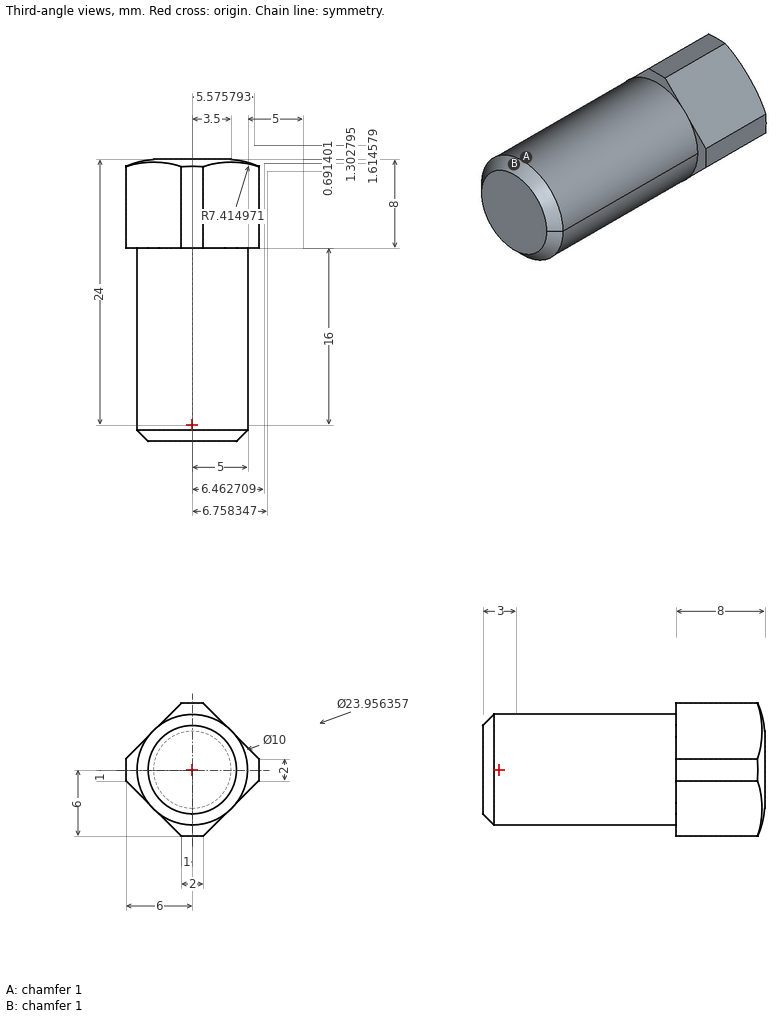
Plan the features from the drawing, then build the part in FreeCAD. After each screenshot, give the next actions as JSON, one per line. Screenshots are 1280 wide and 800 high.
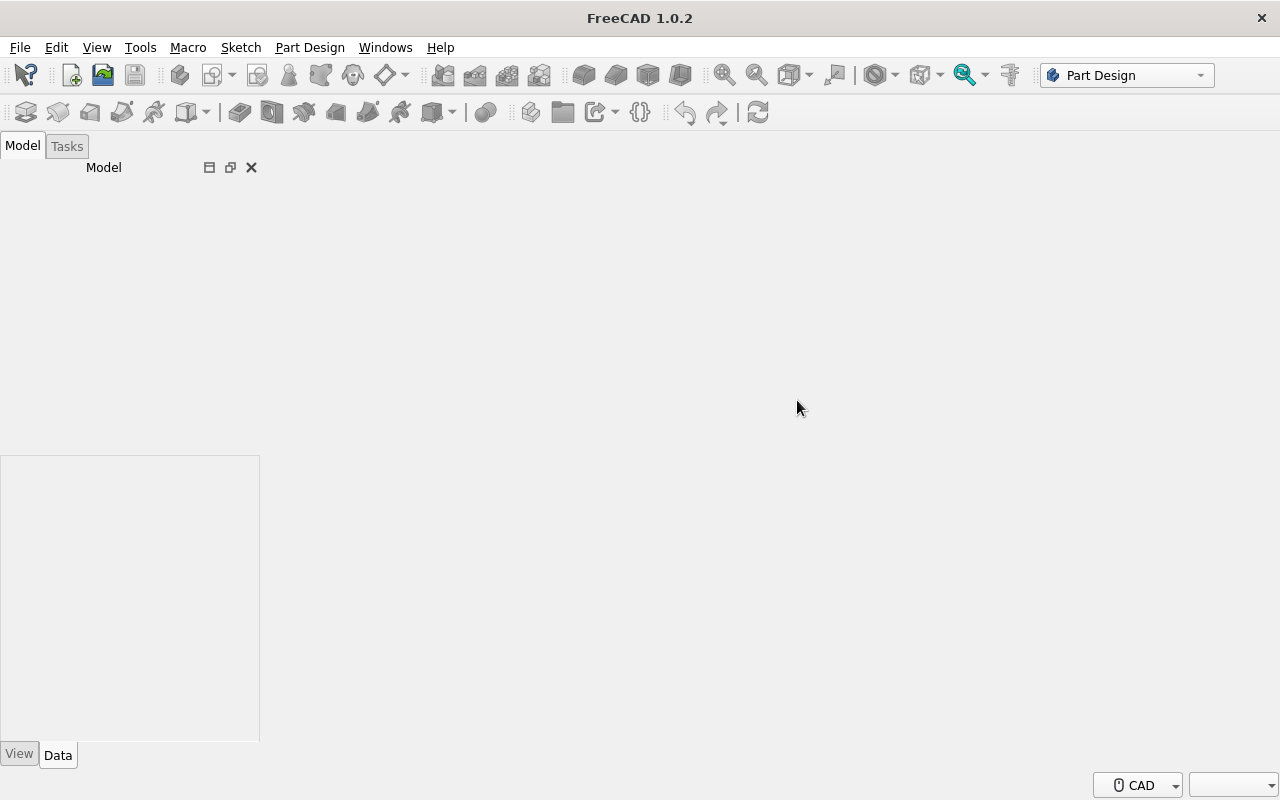
{"action": "key", "text": "ctrl+n"}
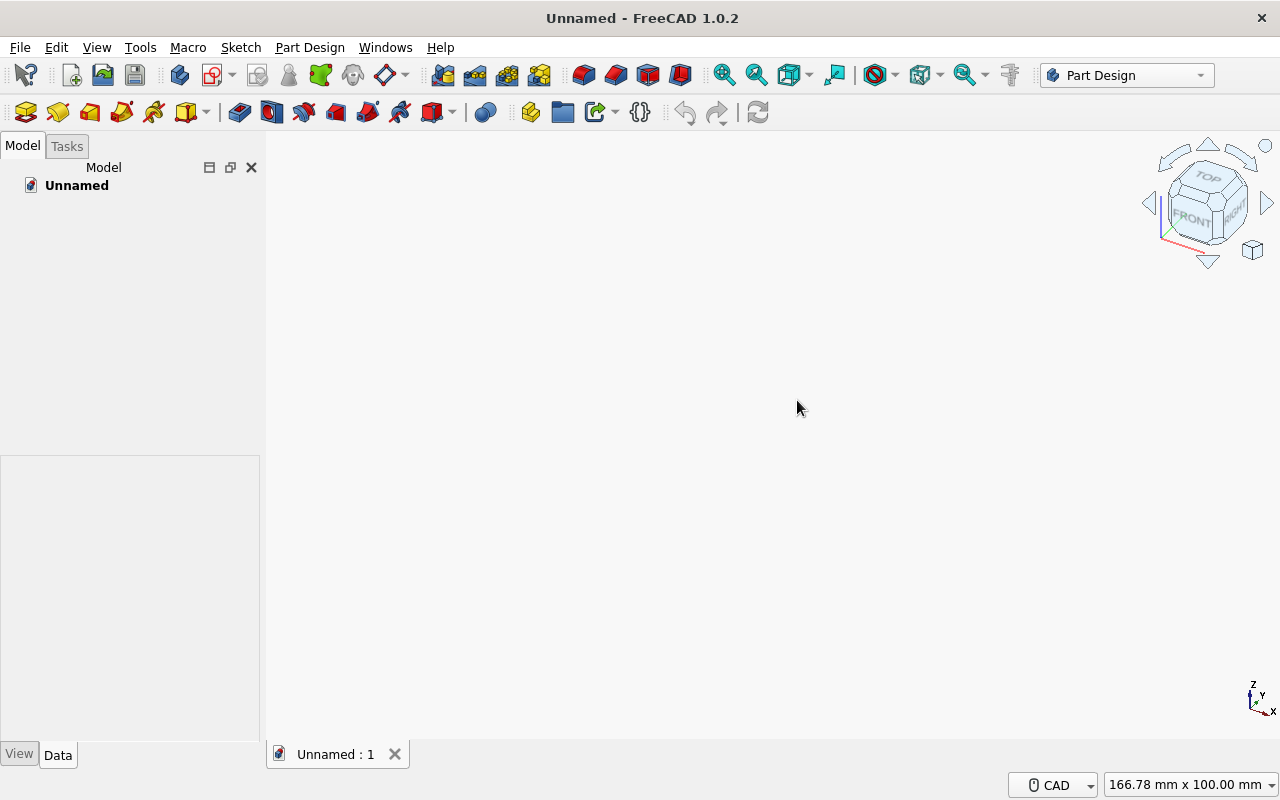
{"action": "left_click", "coordinate": [212, 76]}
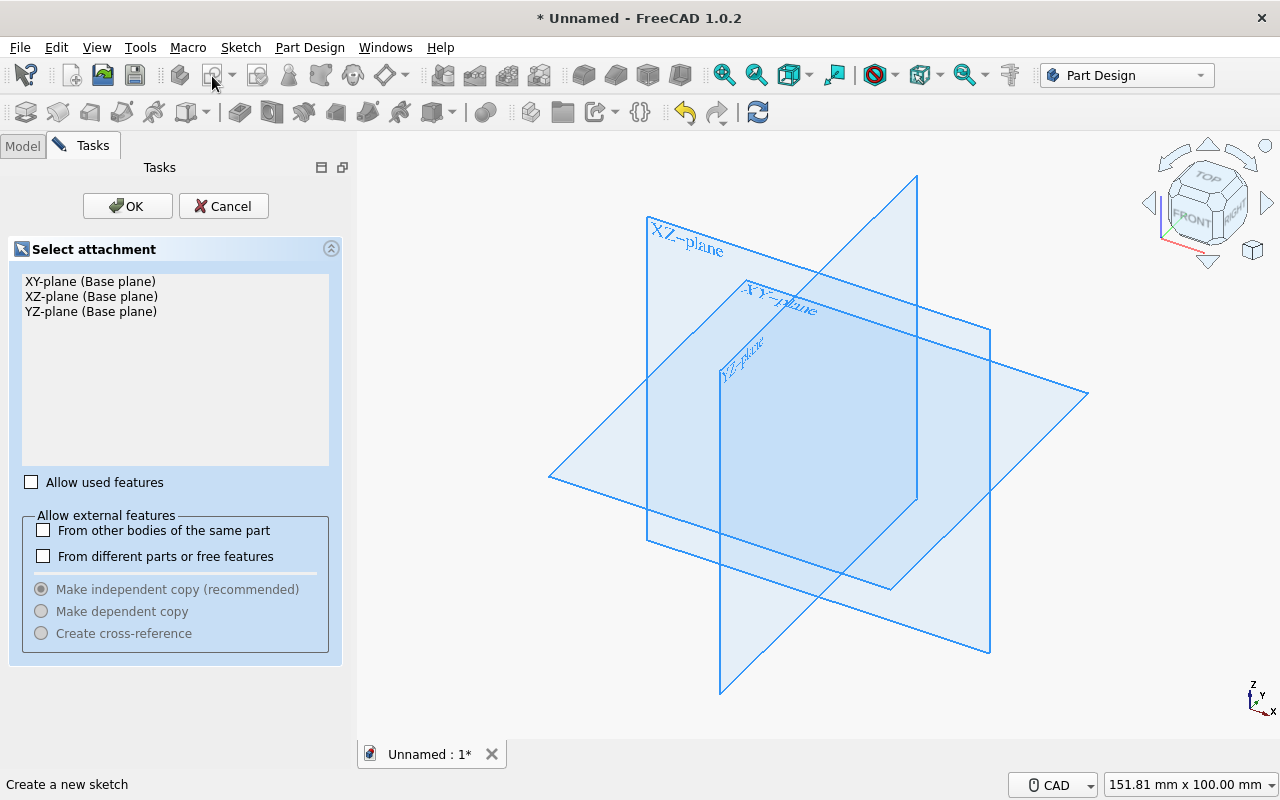
{"action": "left_click", "coordinate": [82, 282]}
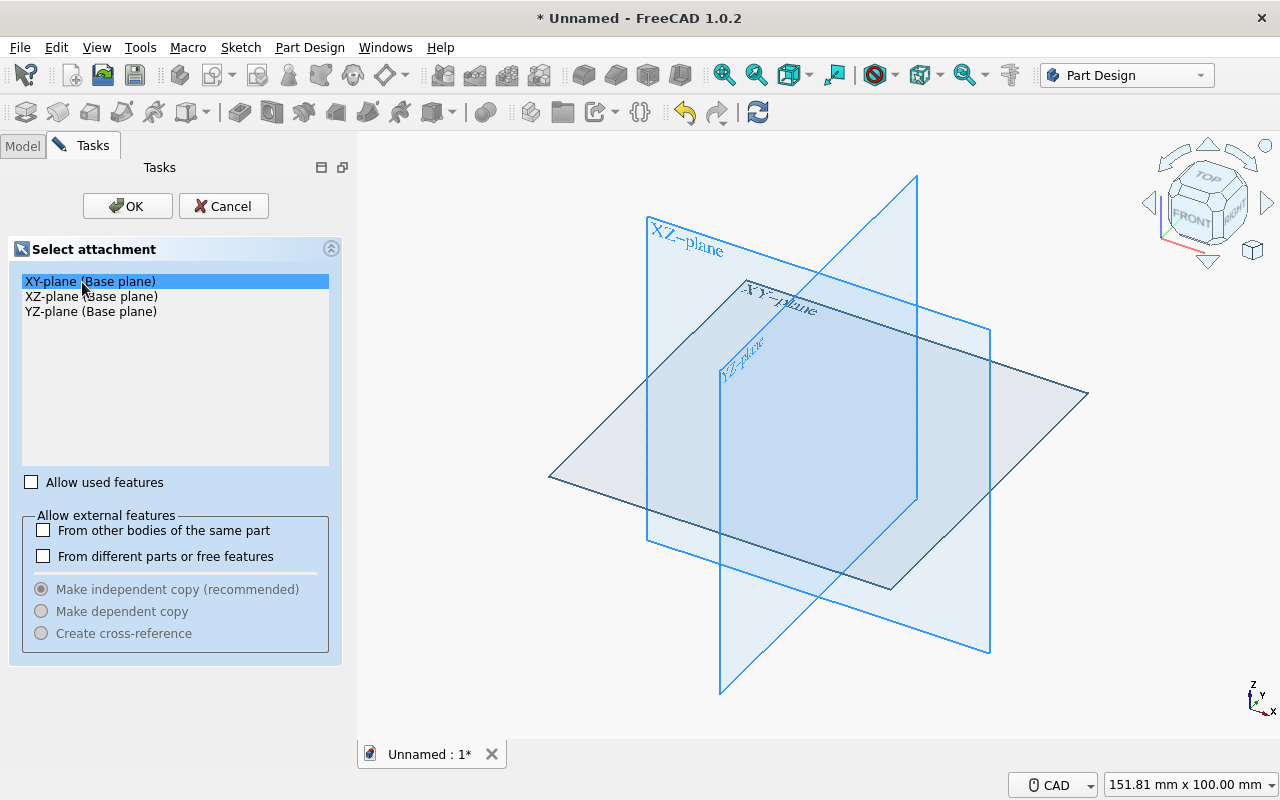
{"action": "left_click", "coordinate": [128, 206]}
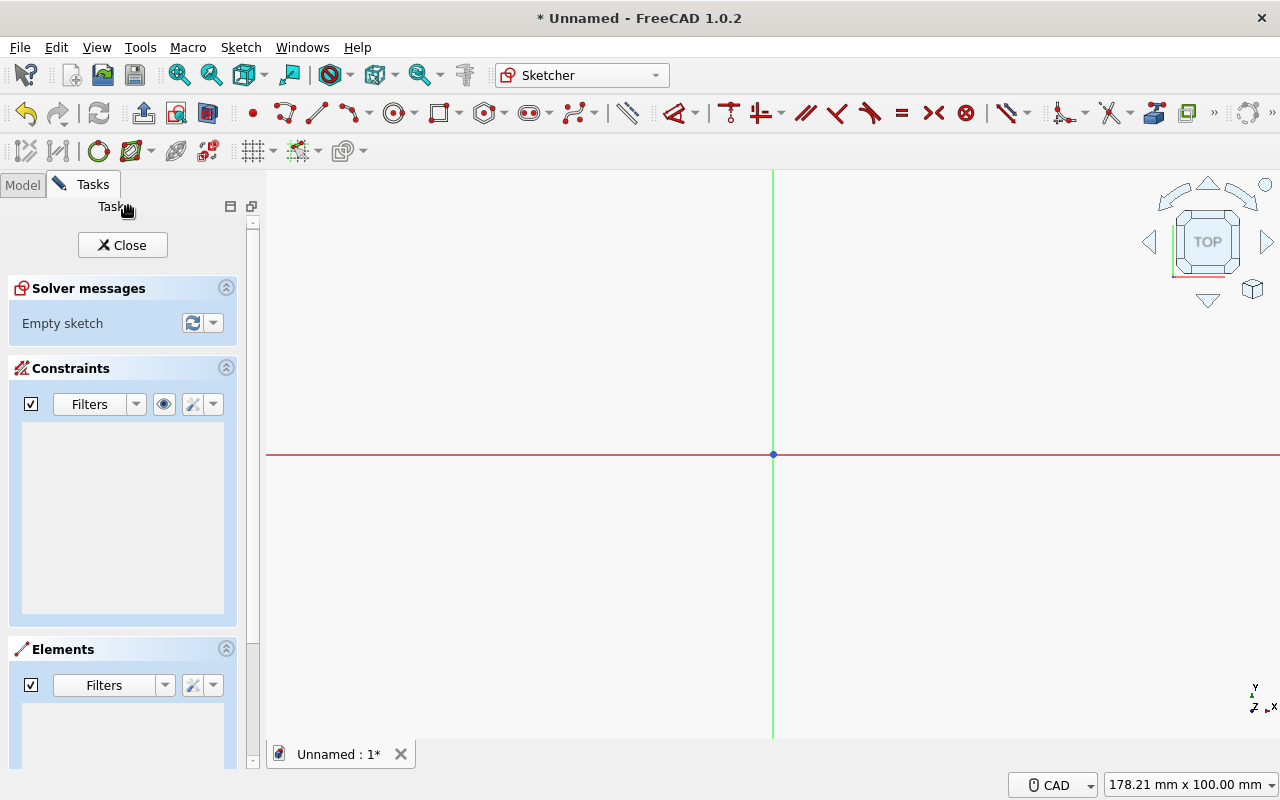
{"action": "scroll", "coordinate": [858, 346], "scroll_direction": "up", "scroll_amount": 5}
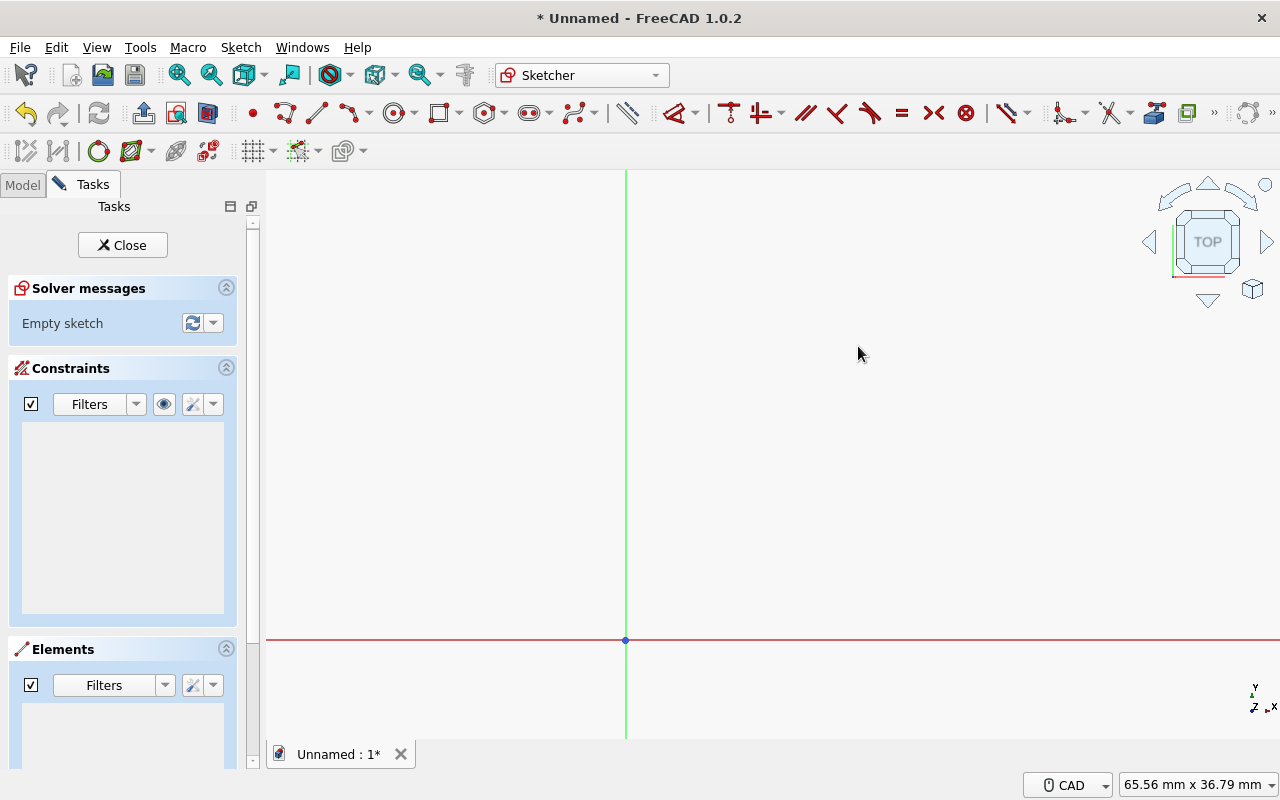
{"action": "left_click", "coordinate": [286, 114]}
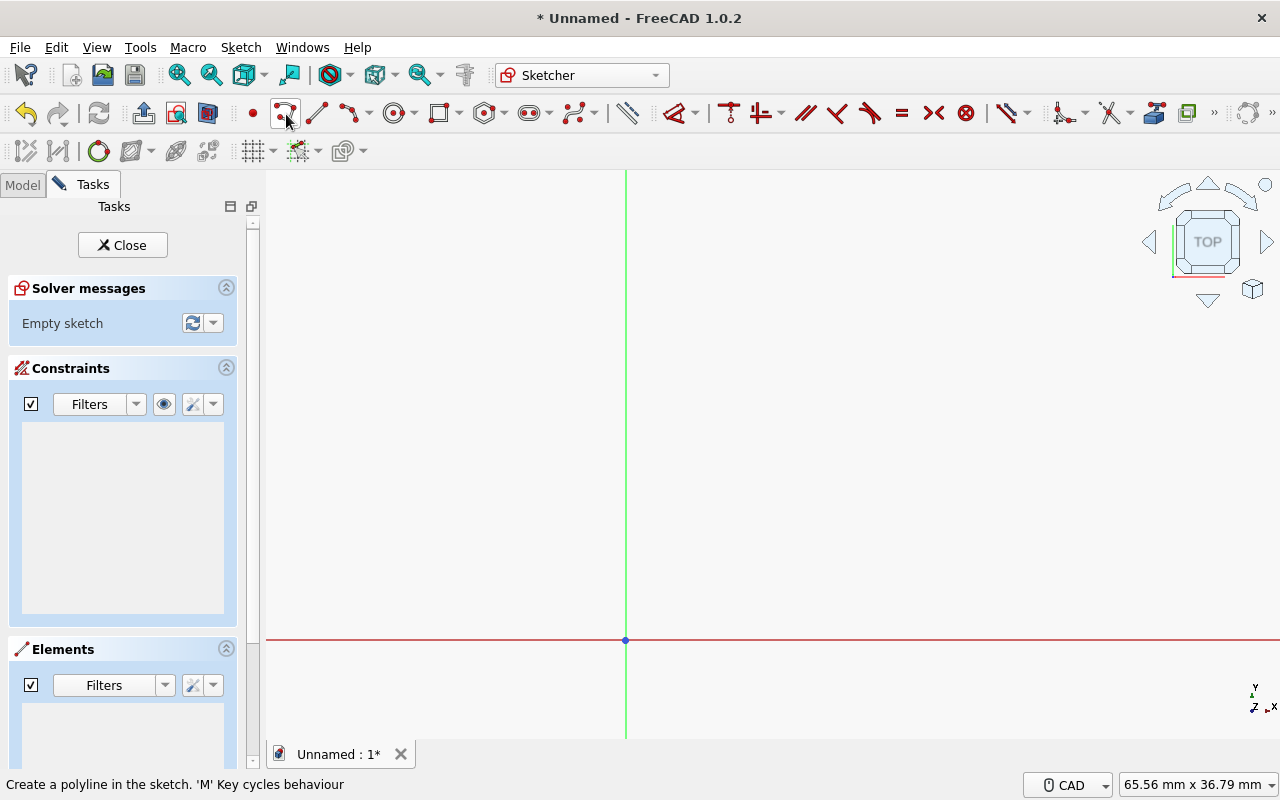
{"action": "left_click", "coordinate": [626, 640]}
{"action": "left_click", "coordinate": [703, 631]}
{"action": "left_click", "coordinate": [703, 393]}
{"action": "left_click", "coordinate": [781, 393]}
{"action": "left_click", "coordinate": [781, 269]}
{"action": "left_click", "coordinate": [635, 269]}
{"action": "left_click", "coordinate": [626, 640]}
{"action": "key", "text": "Escape"}
{"action": "key", "text": "Escape"}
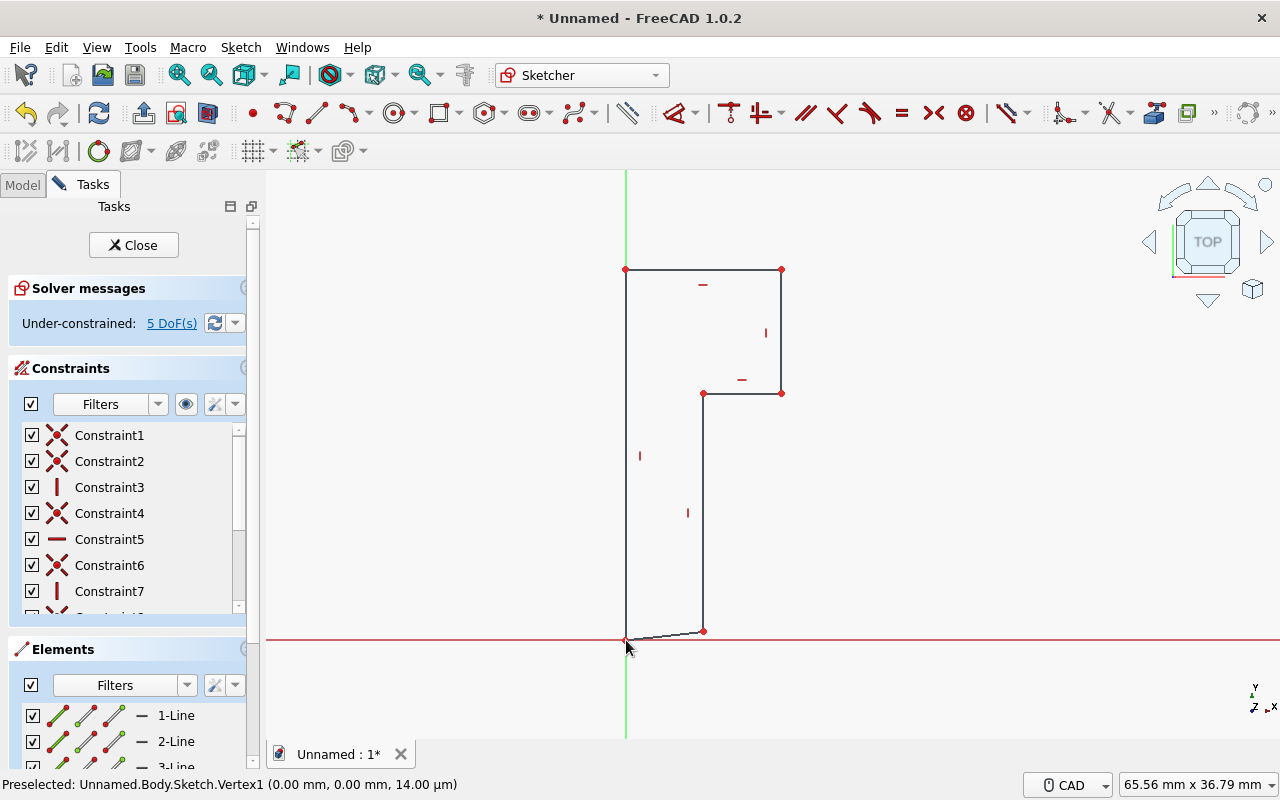
{"action": "left_click", "coordinate": [649, 638]}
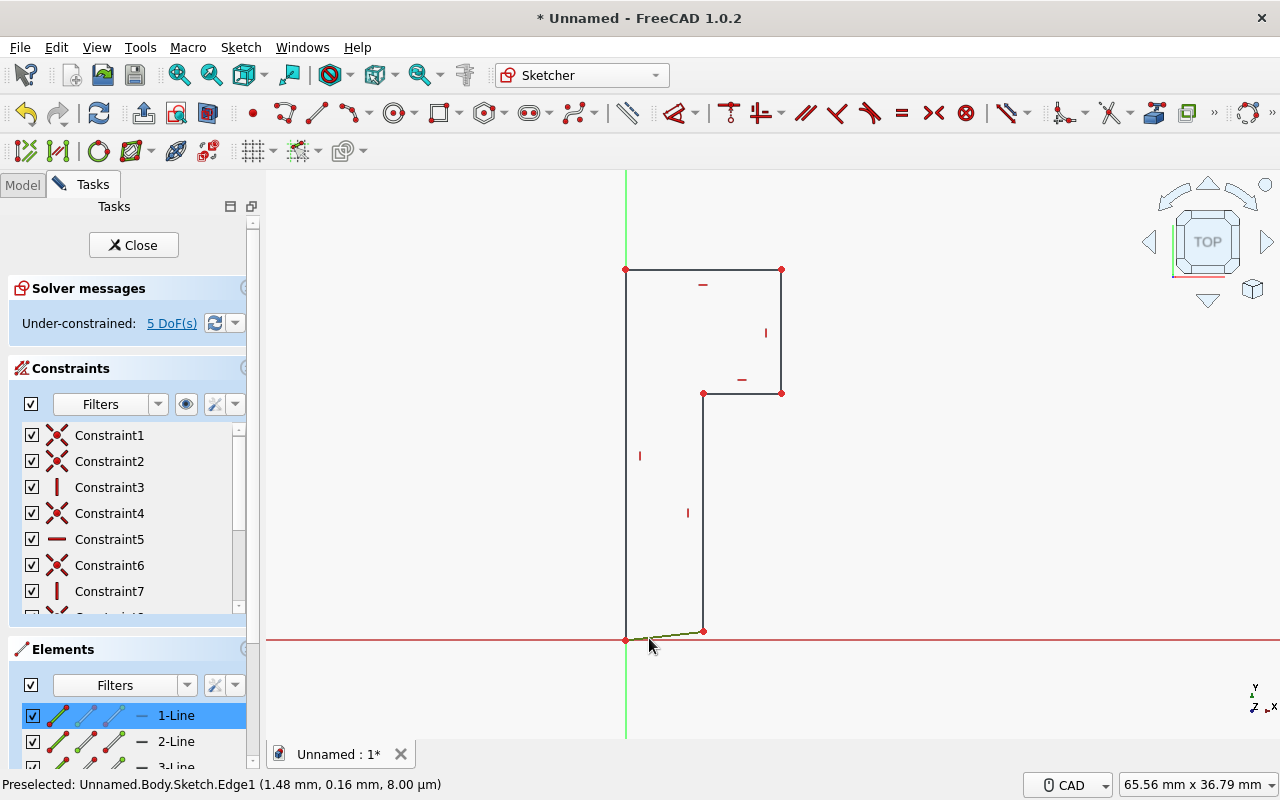
{"action": "key", "text": "h"}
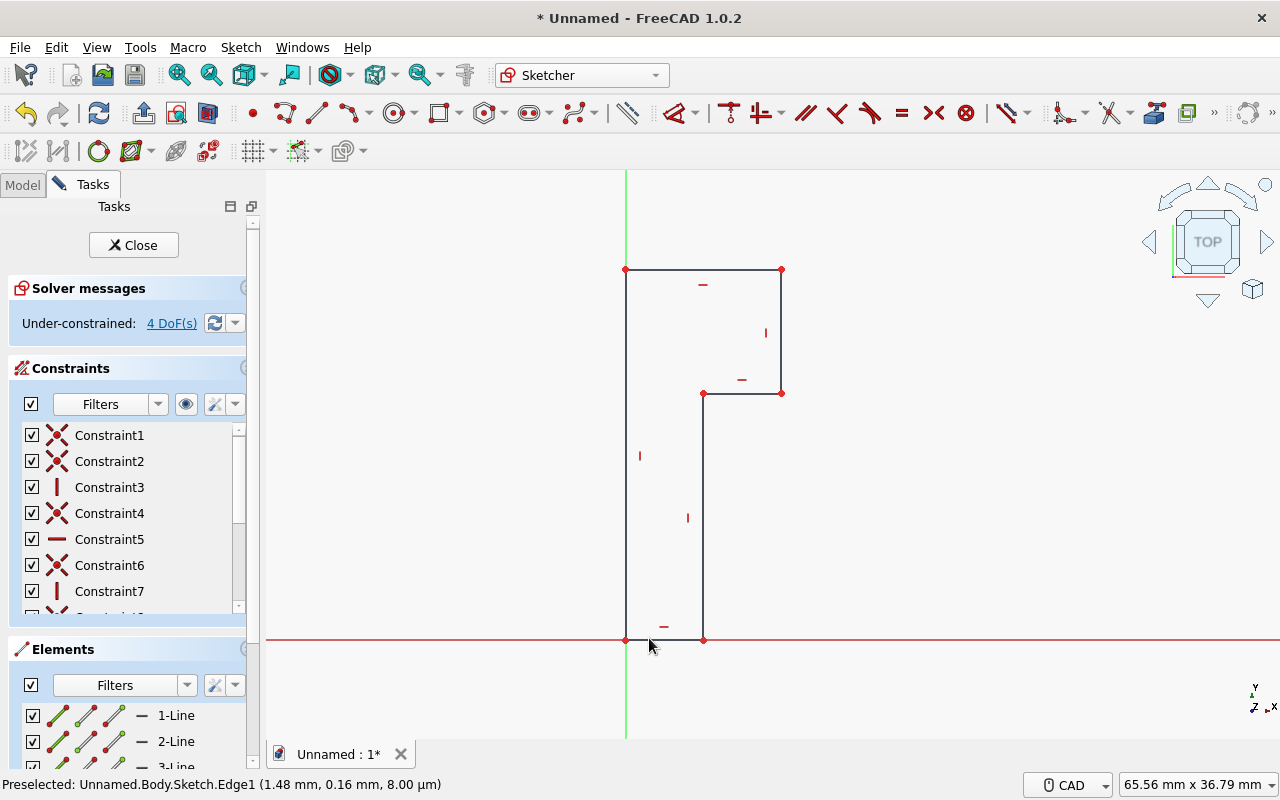
{"action": "left_click", "coordinate": [649, 640]}